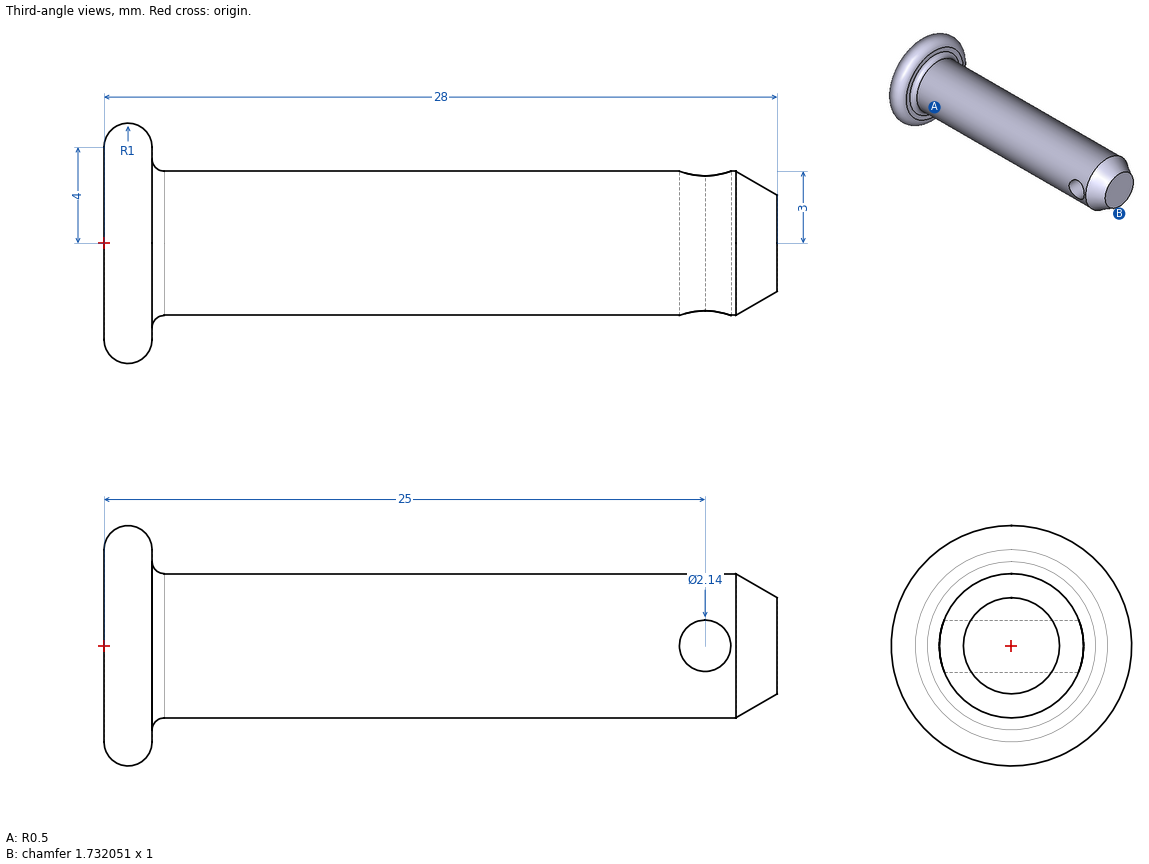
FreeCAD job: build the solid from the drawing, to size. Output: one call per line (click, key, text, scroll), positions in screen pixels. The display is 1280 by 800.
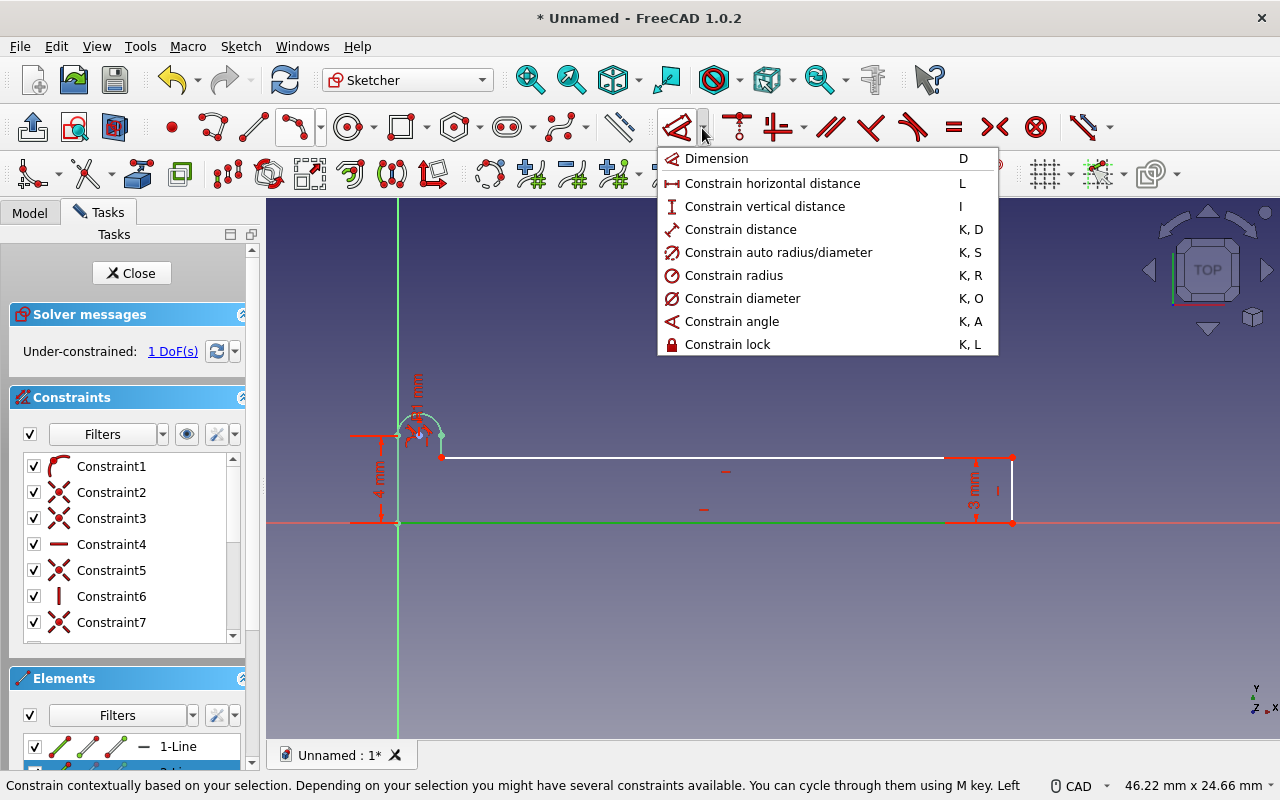
click(828, 184)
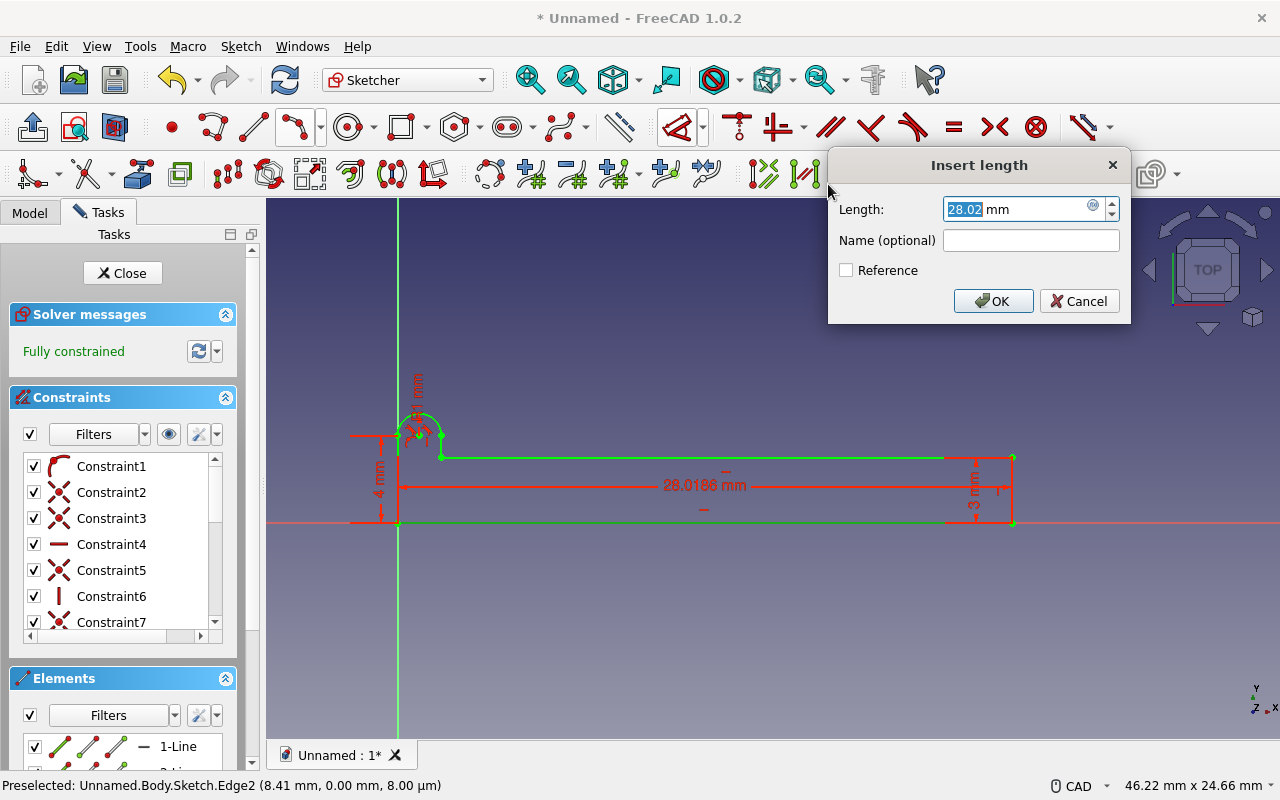
text(28)
key(Return)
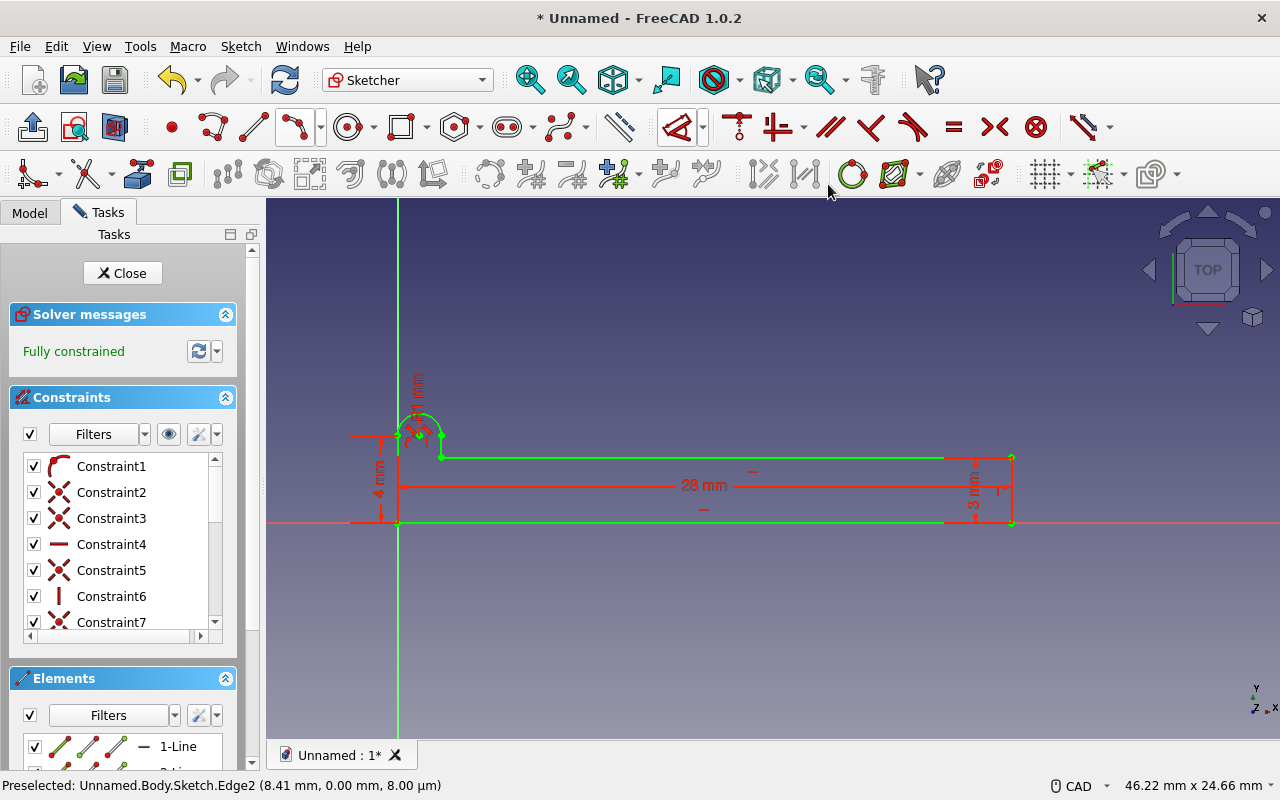
click(123, 273)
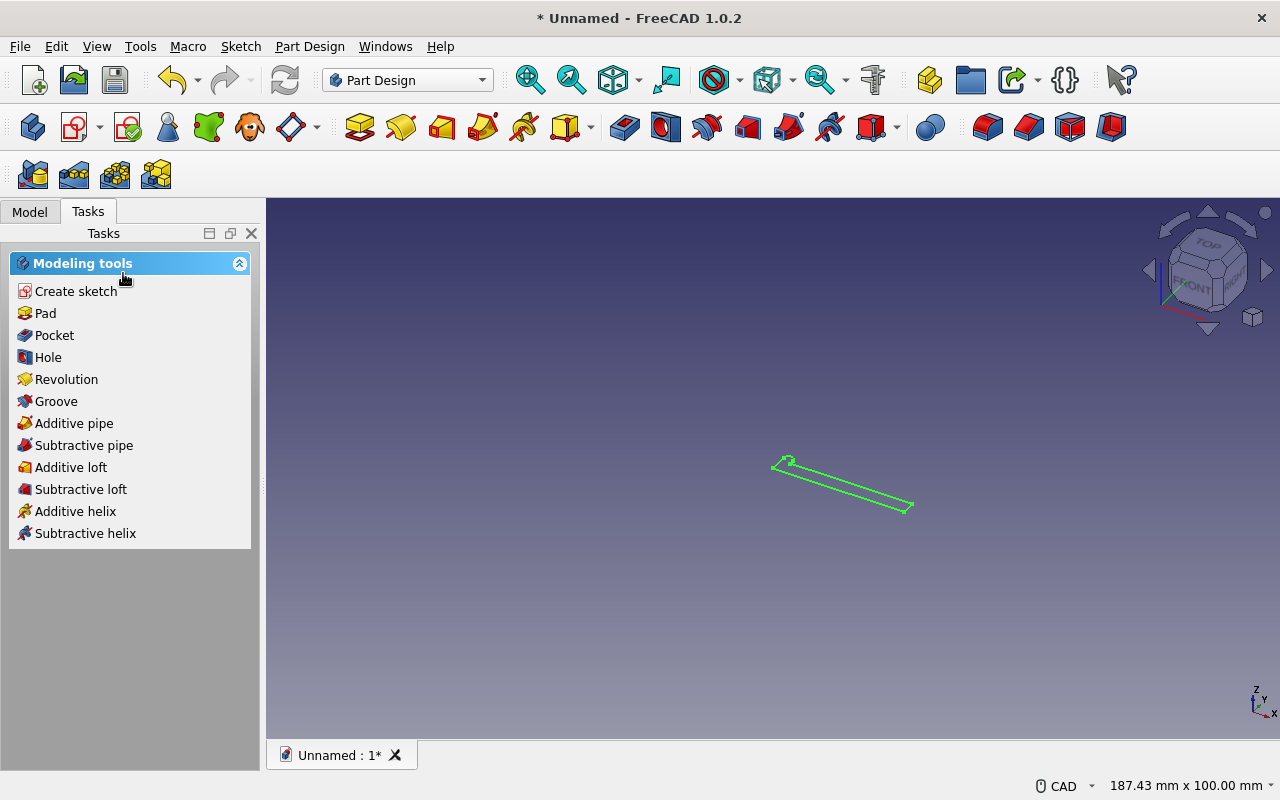
click(401, 128)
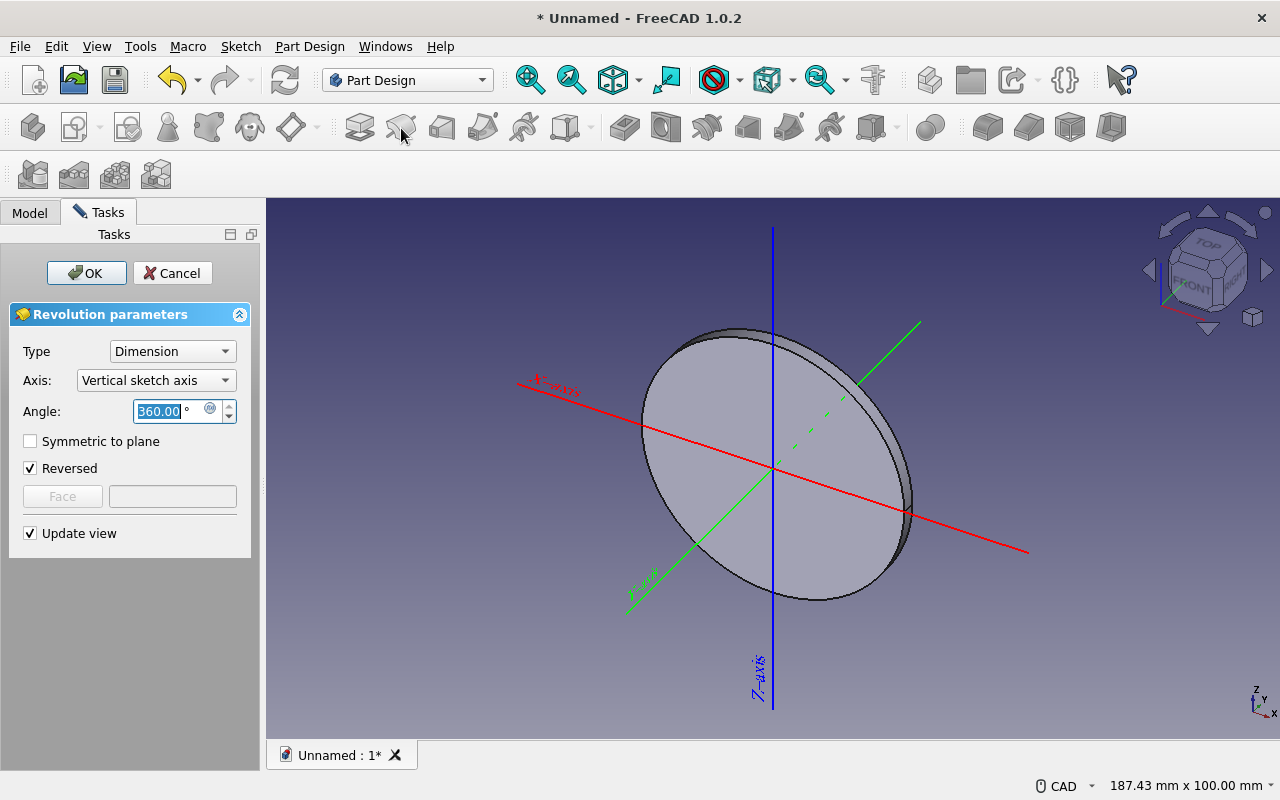
click(157, 380)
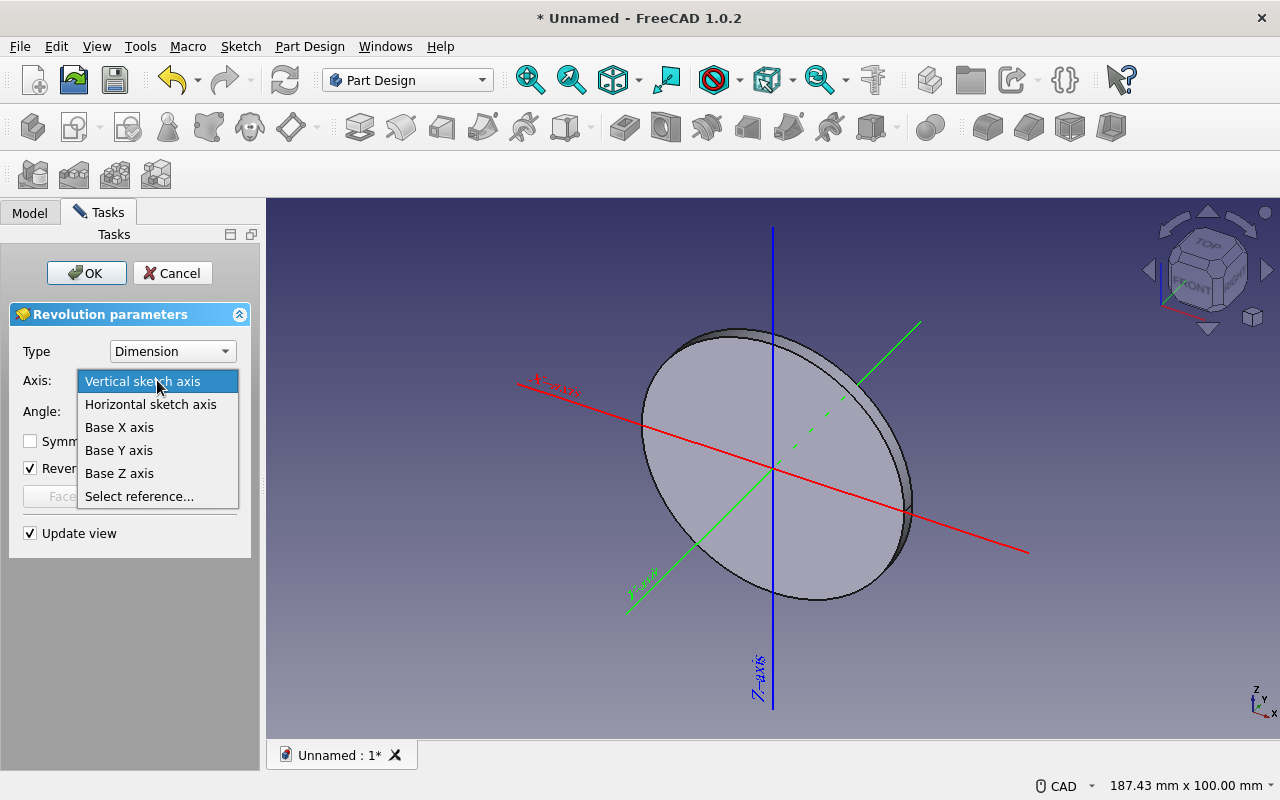
click(156, 404)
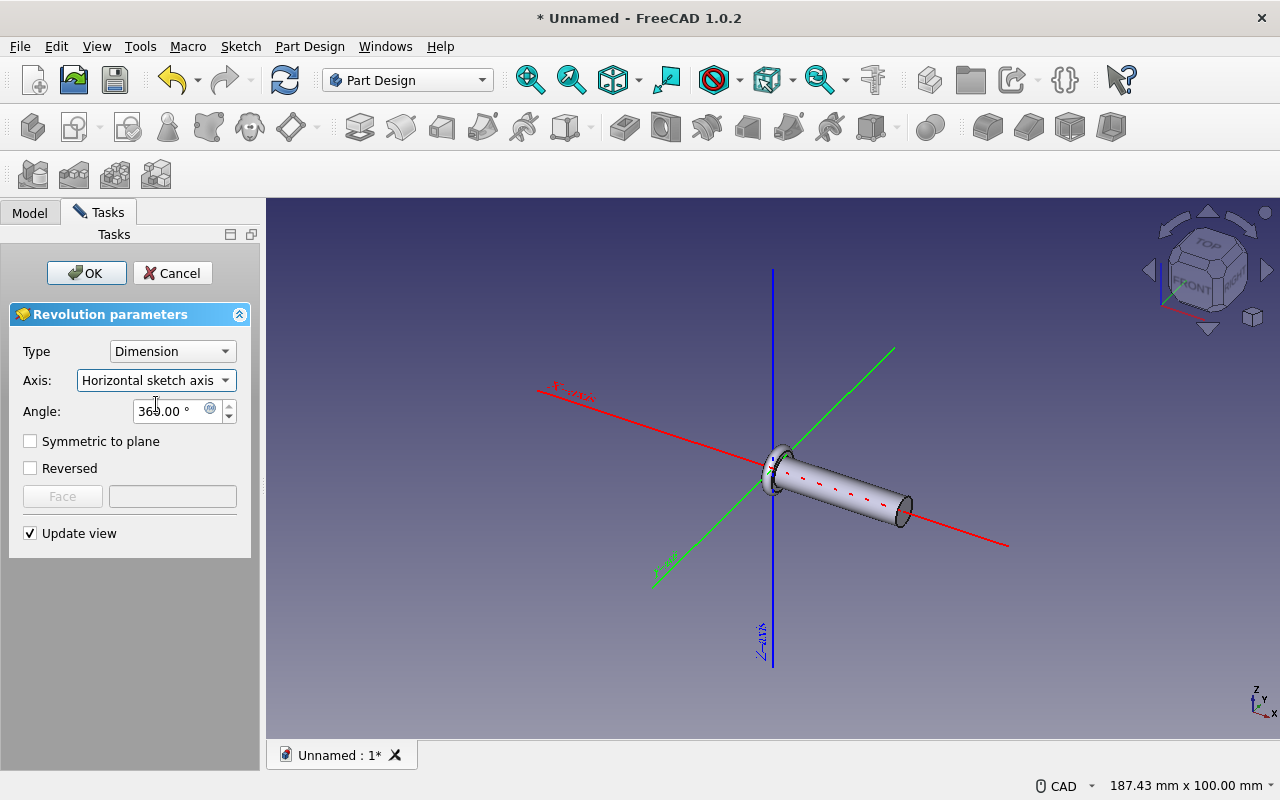
click(87, 273)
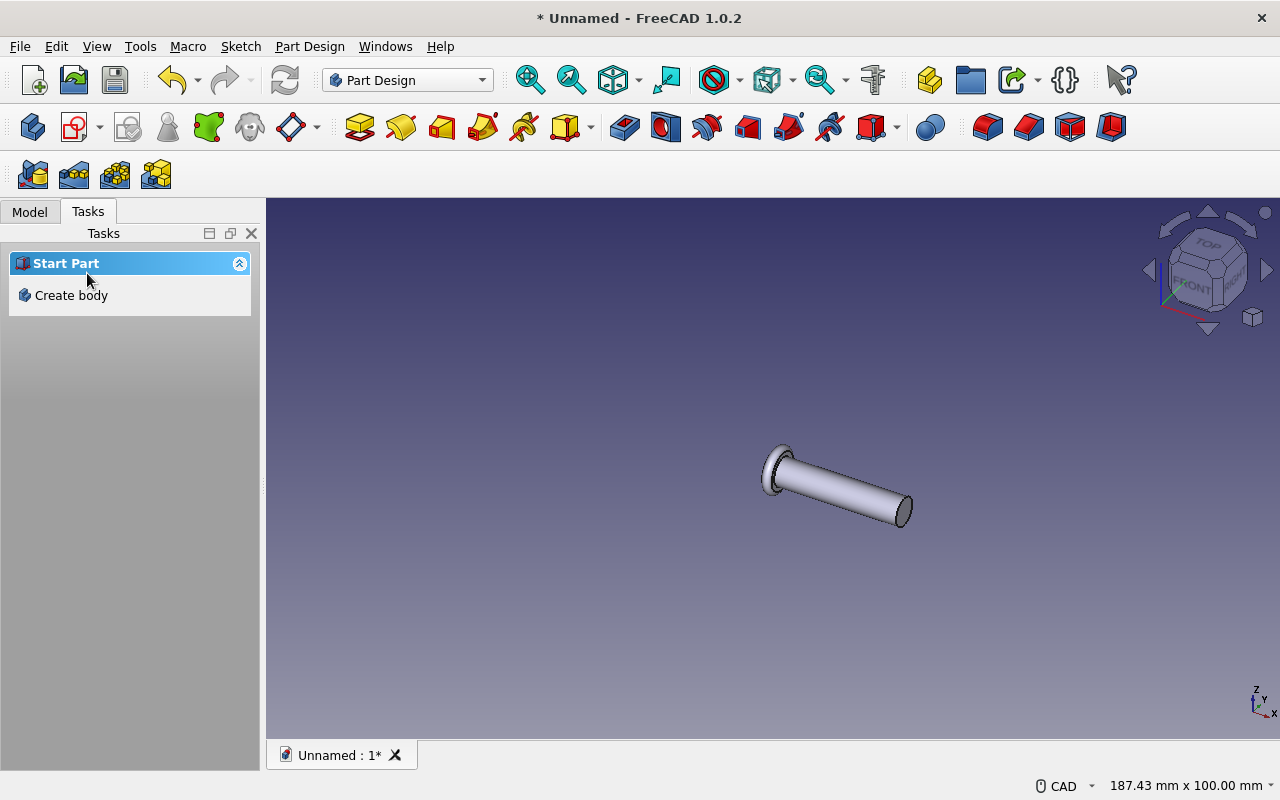
click(531, 80)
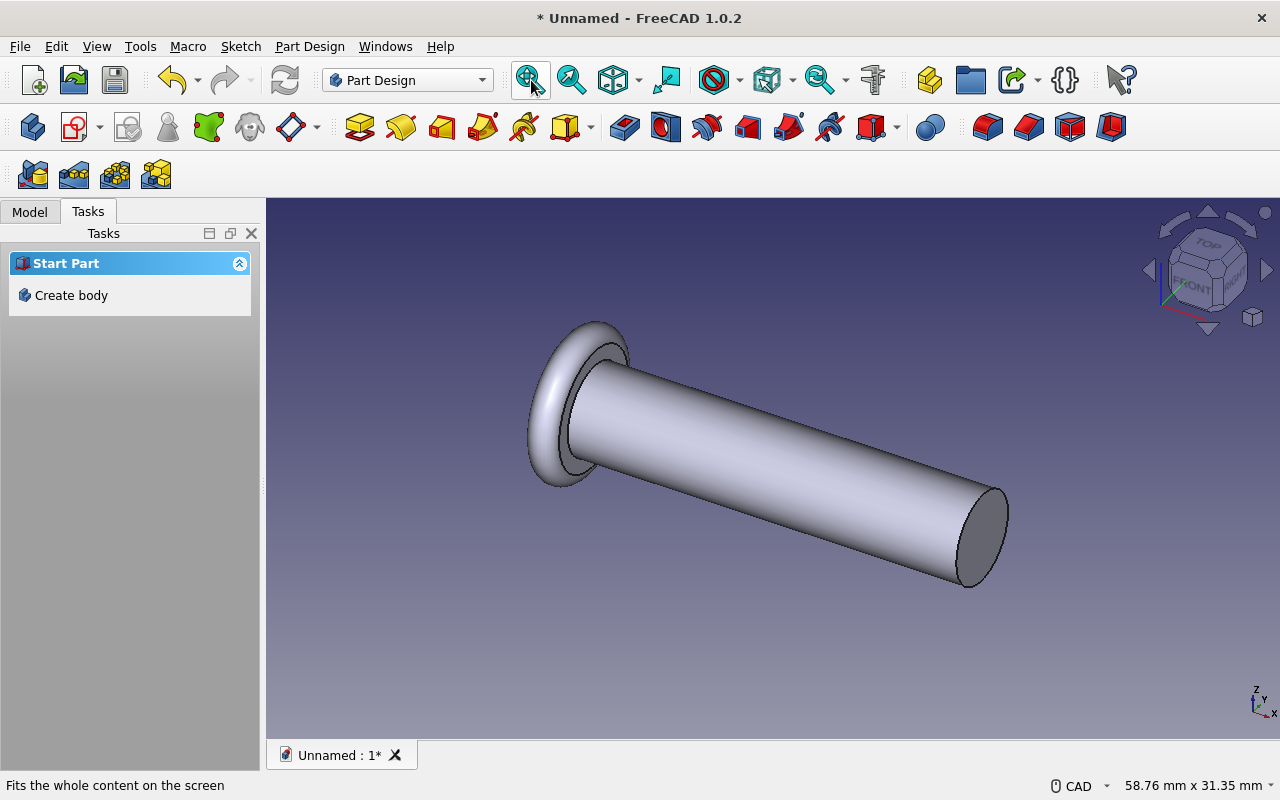
key(0)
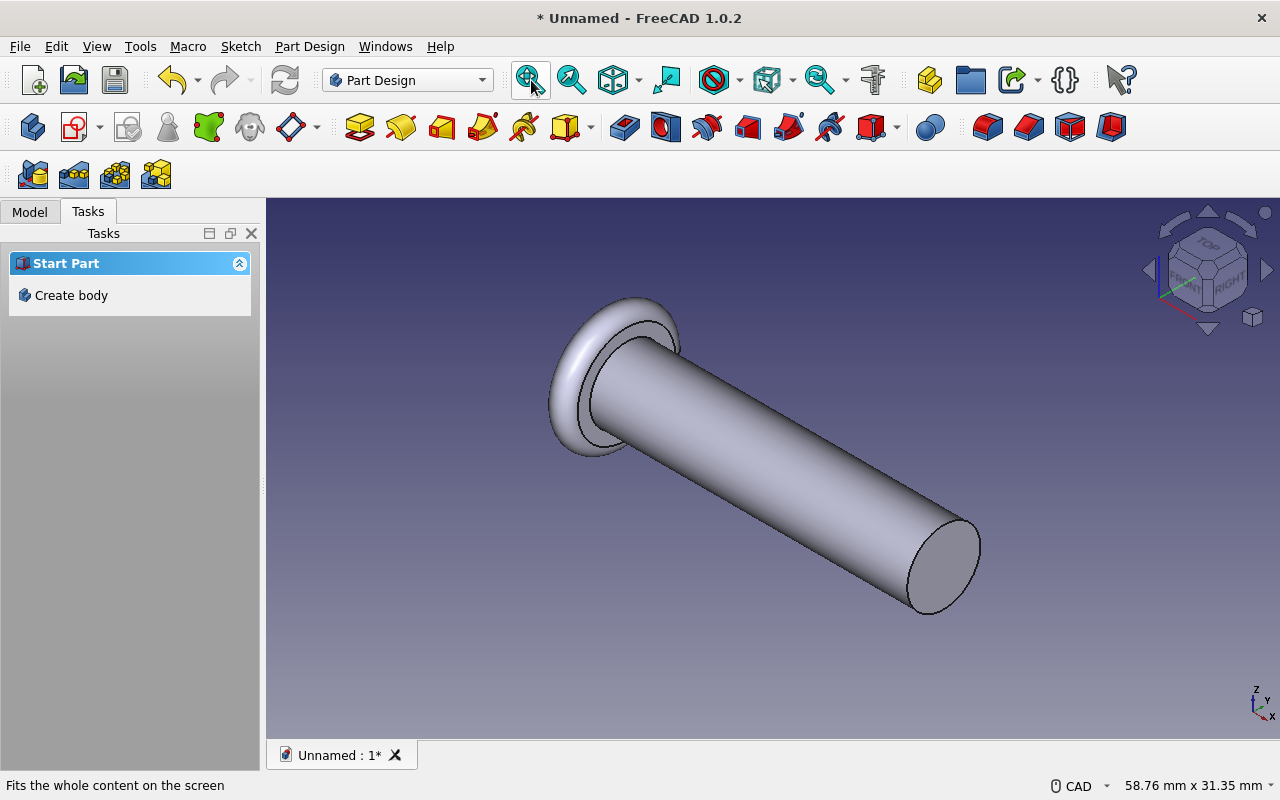
key(2)